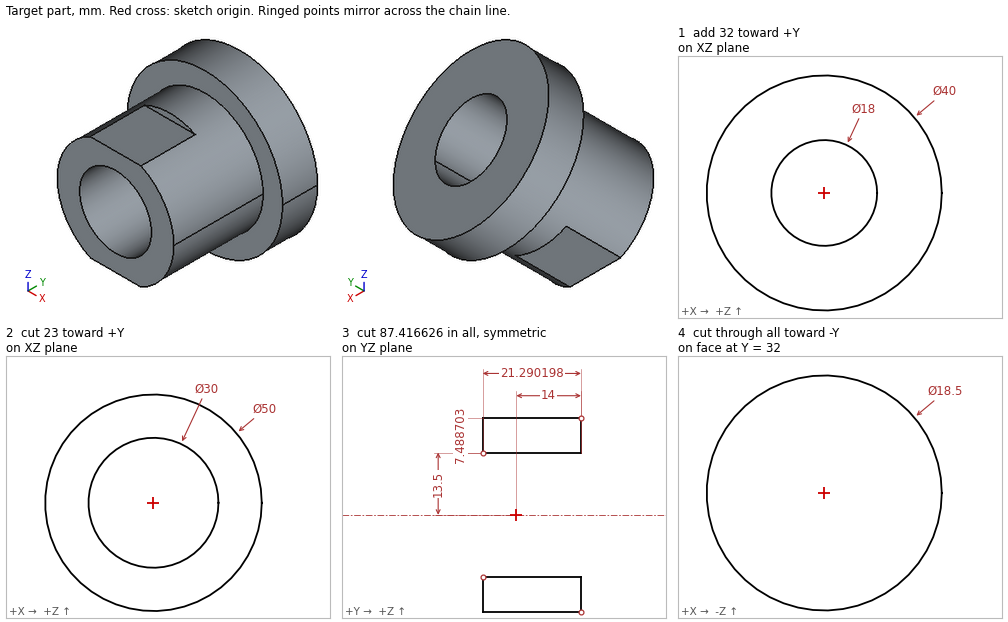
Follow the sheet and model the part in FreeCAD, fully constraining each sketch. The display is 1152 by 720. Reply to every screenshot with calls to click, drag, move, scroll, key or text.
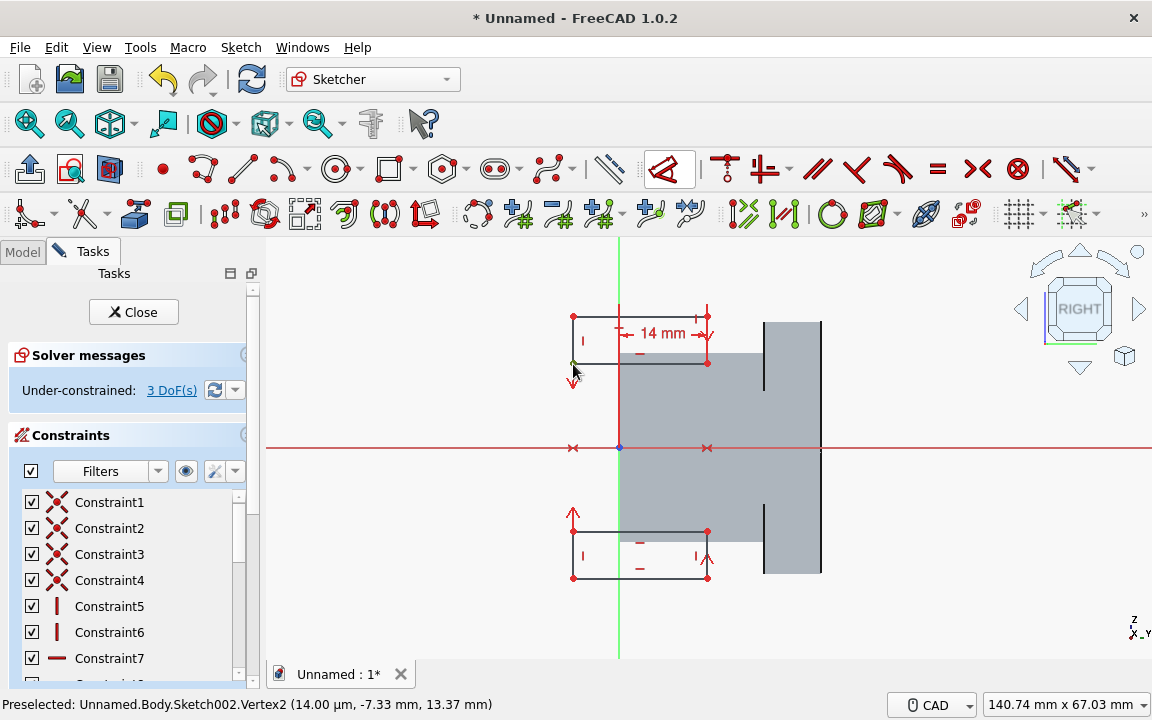
key(i)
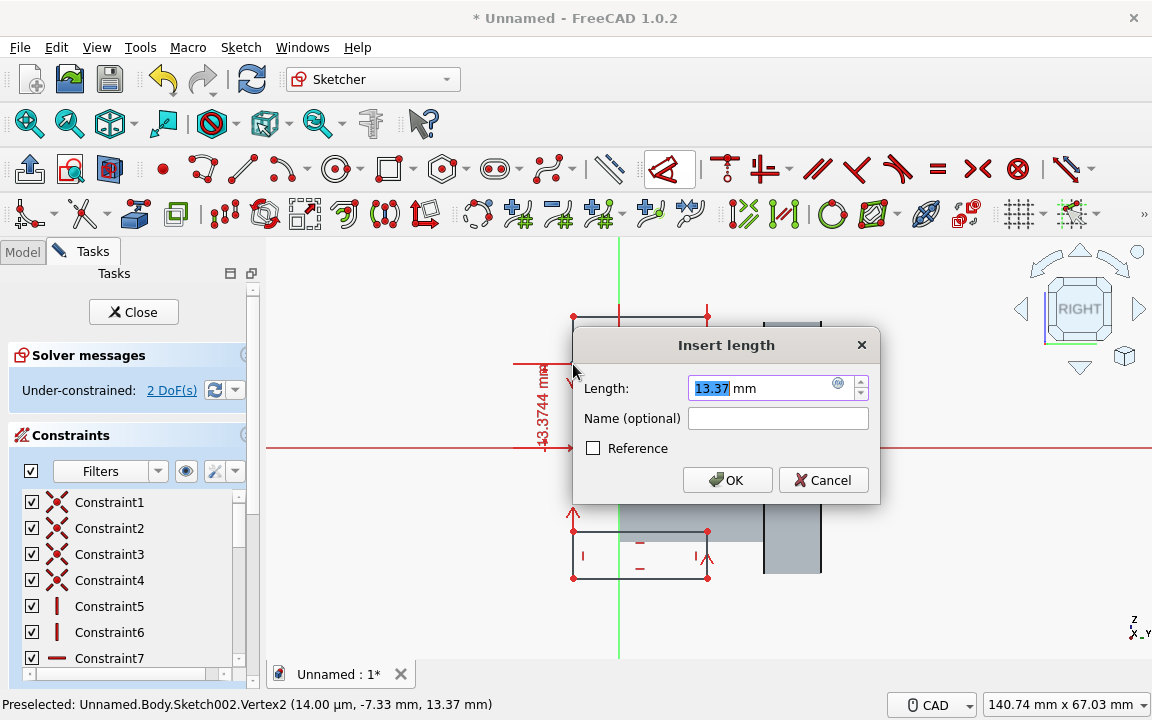
text(13.5)
key(Return)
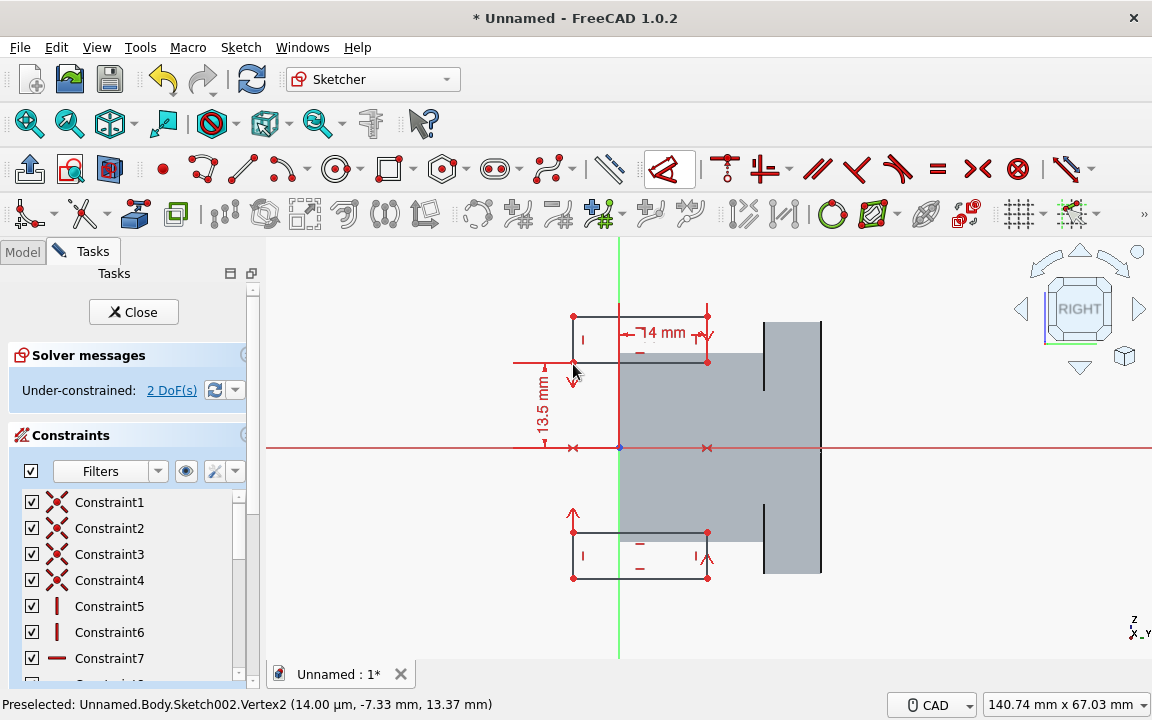
click(573, 330)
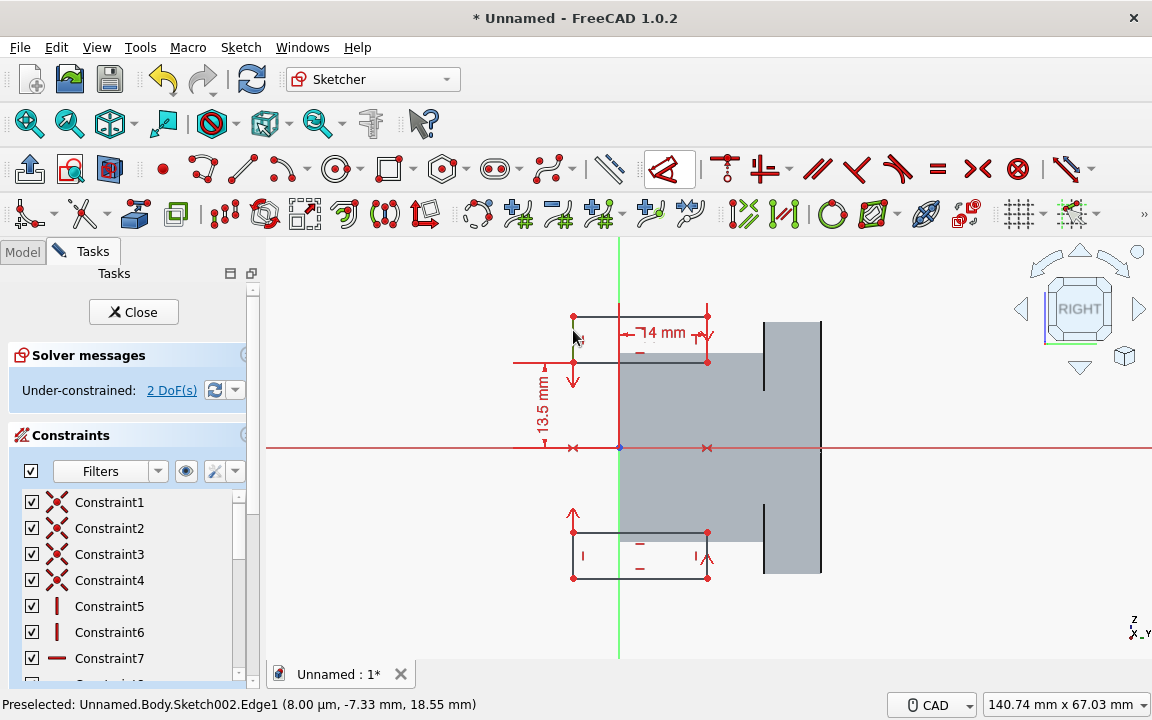
key(i)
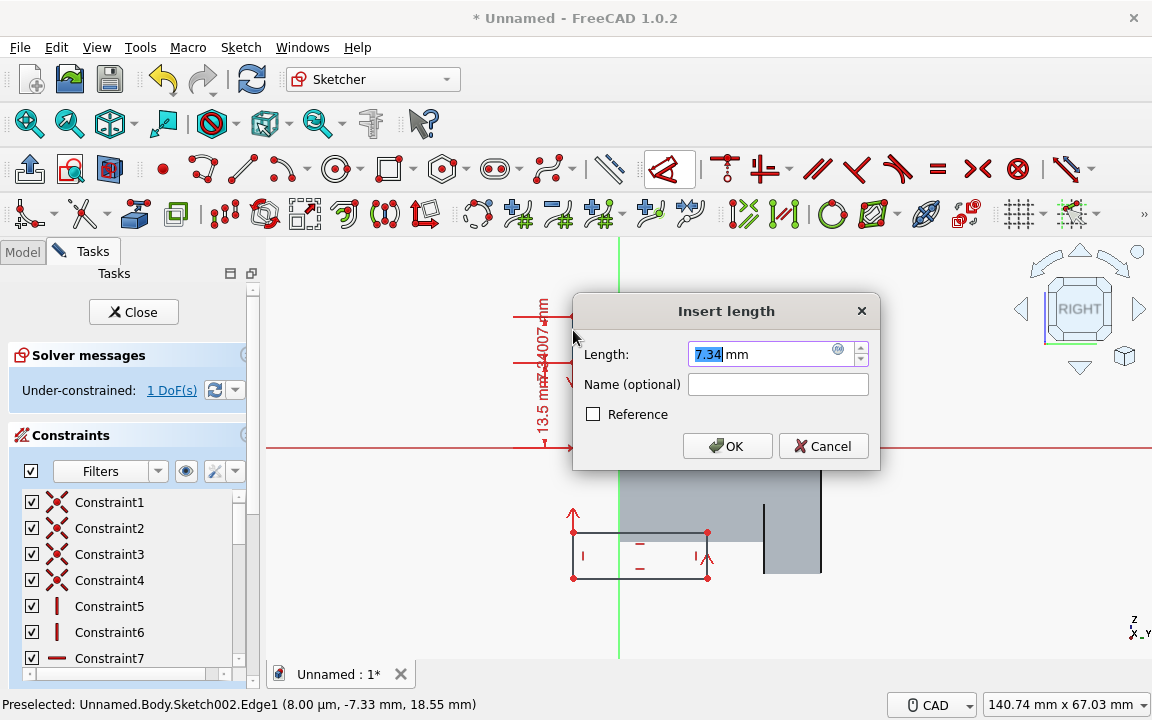
text(7.488703)
key(Return)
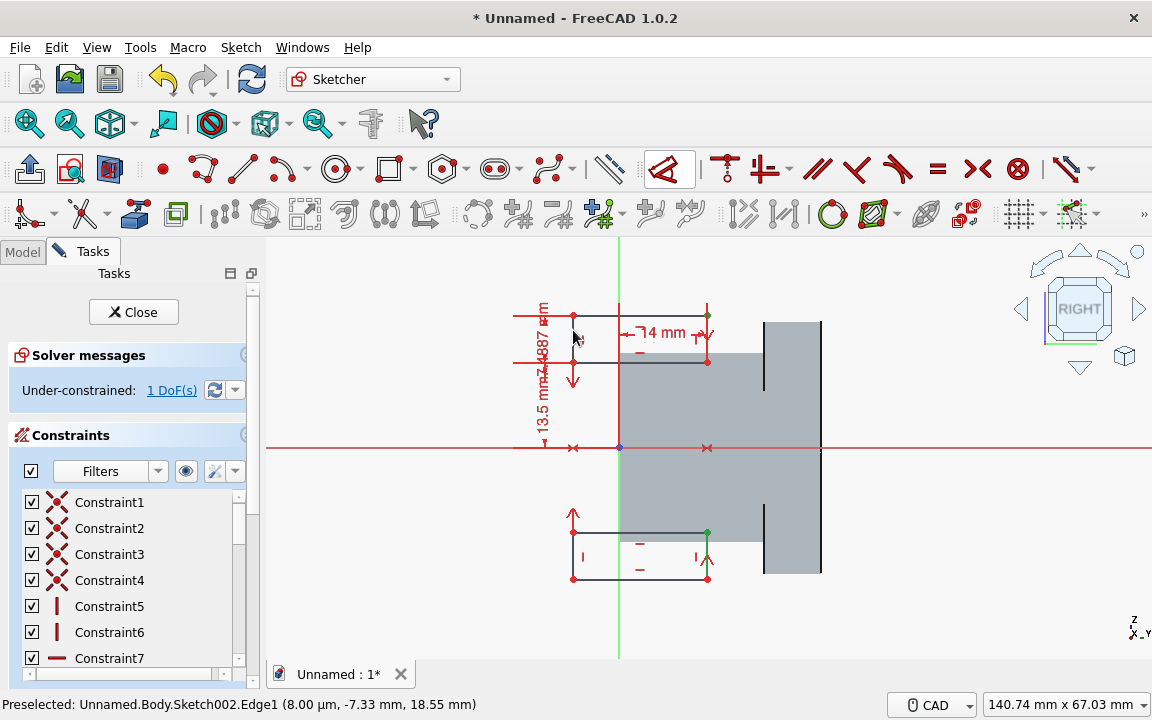
click(667, 363)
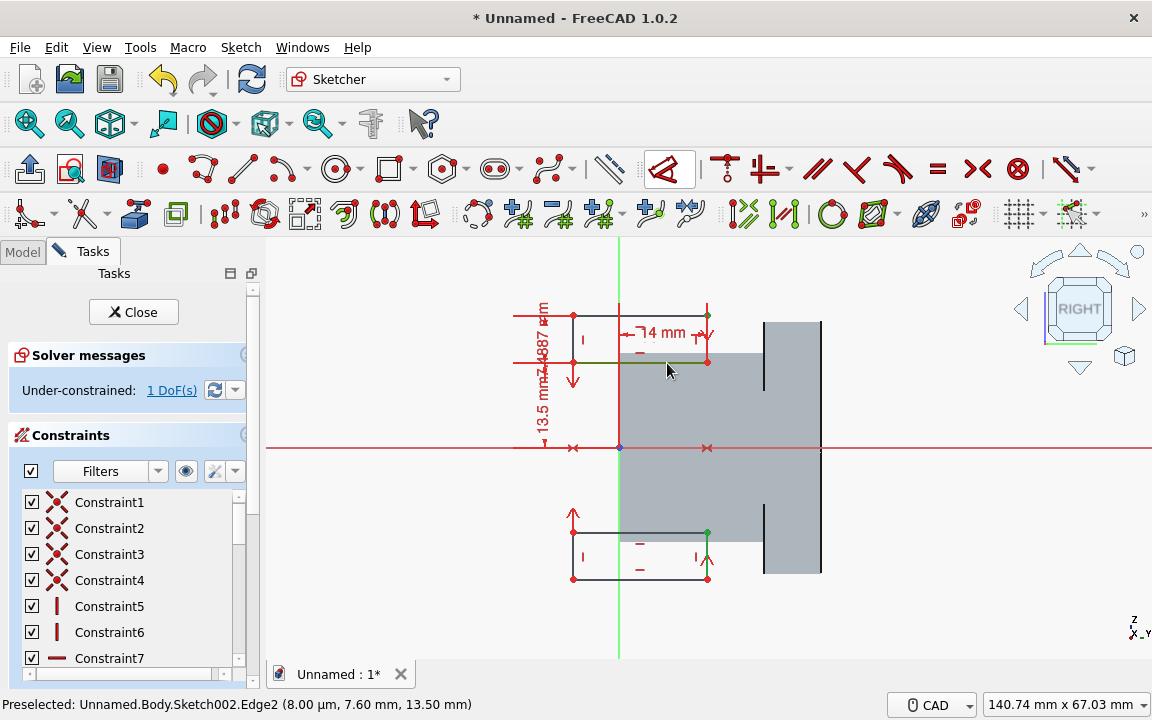
key(l)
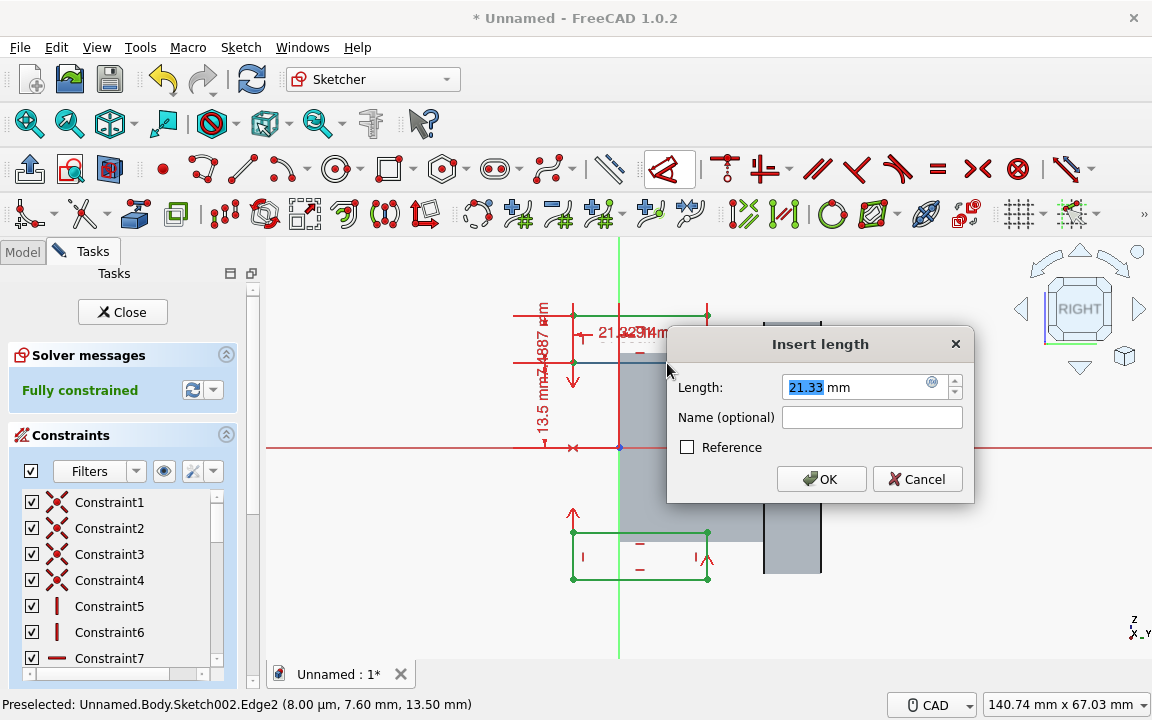
text(21.290198)
key(Return)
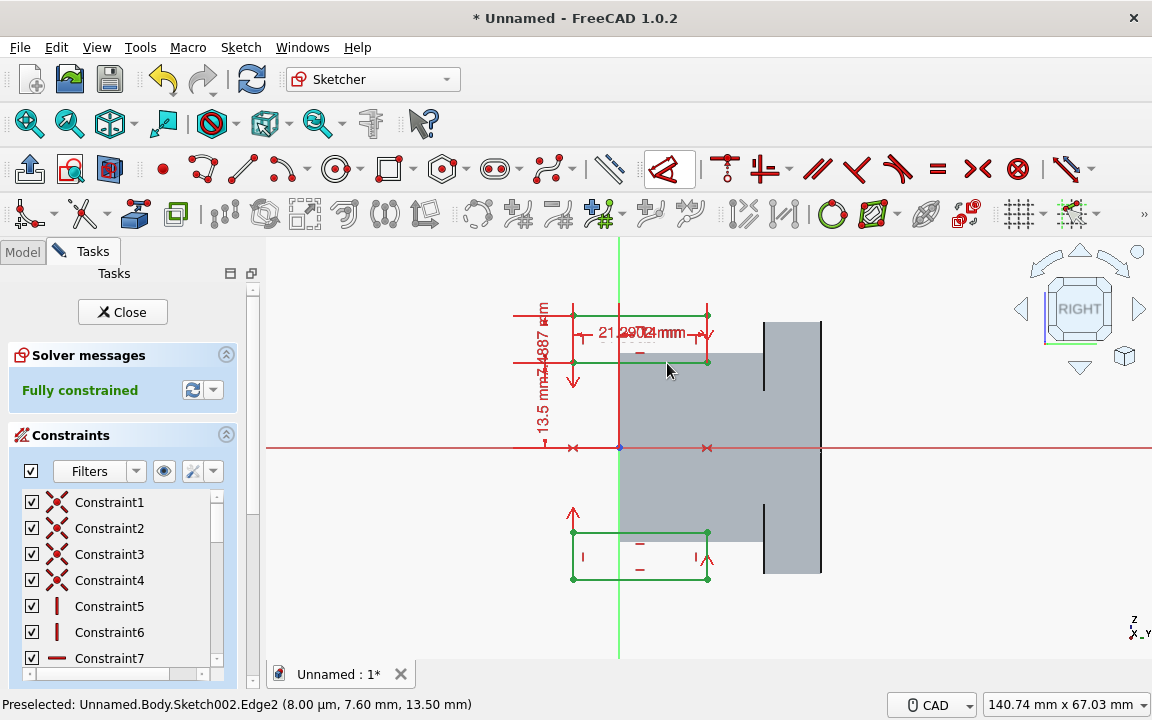
click(123, 312)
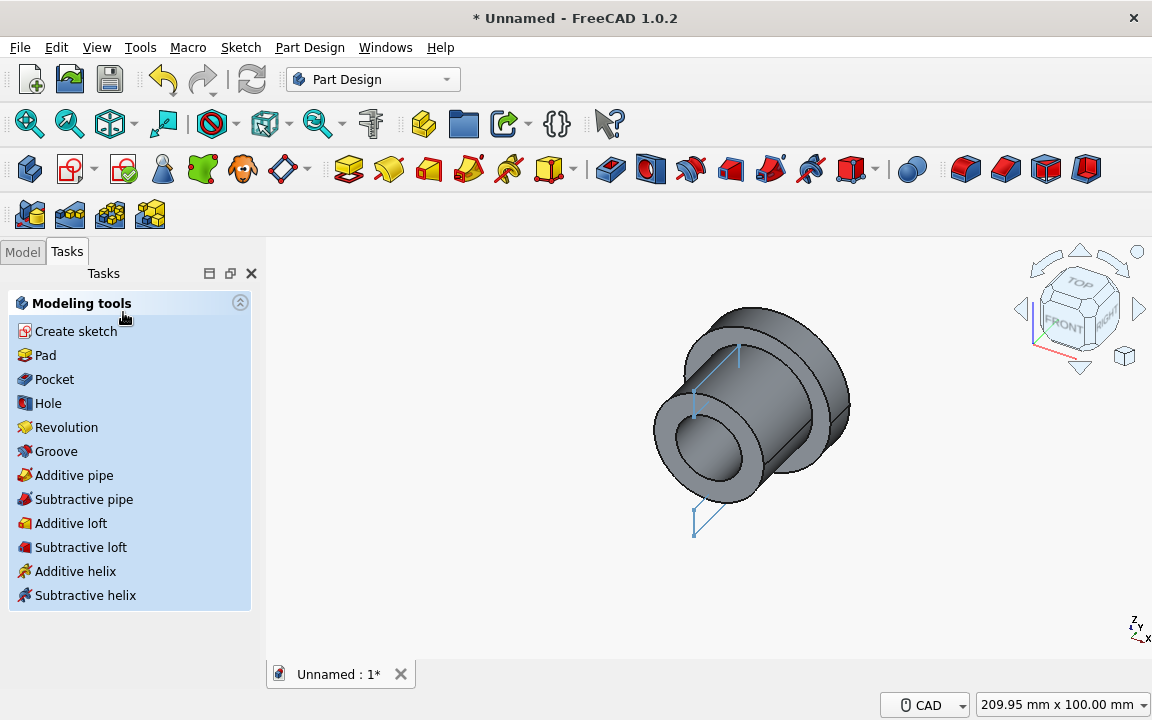
click(612, 170)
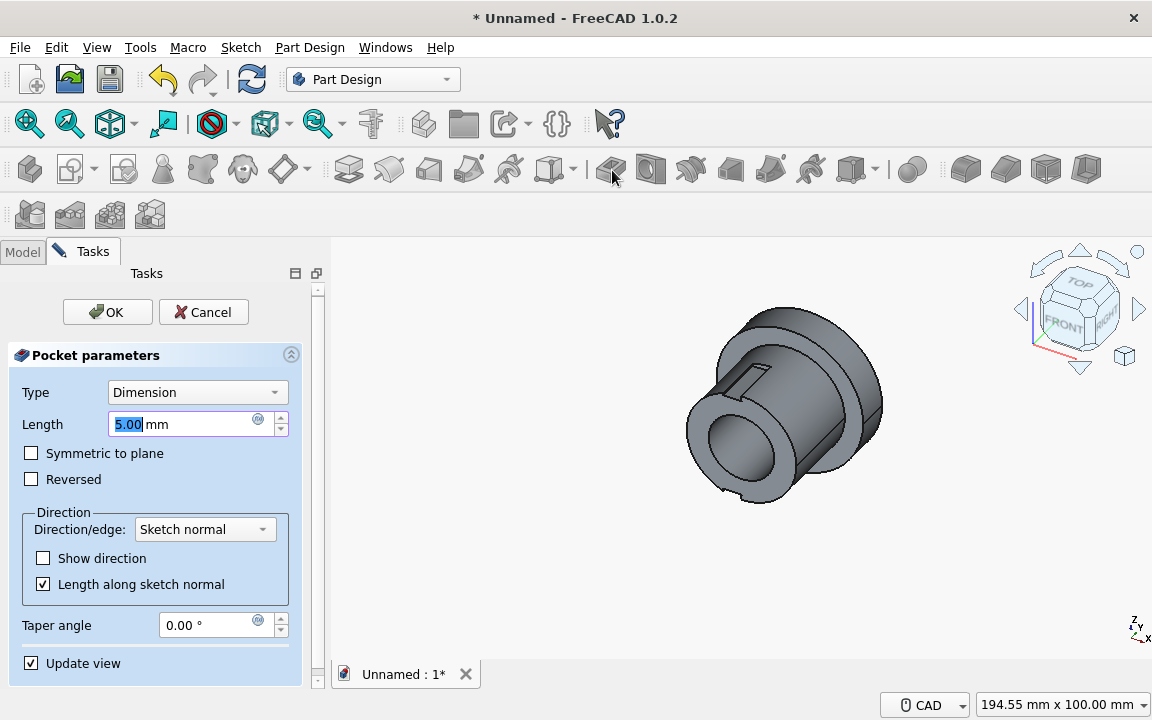
text(87.416626)
key(Tab)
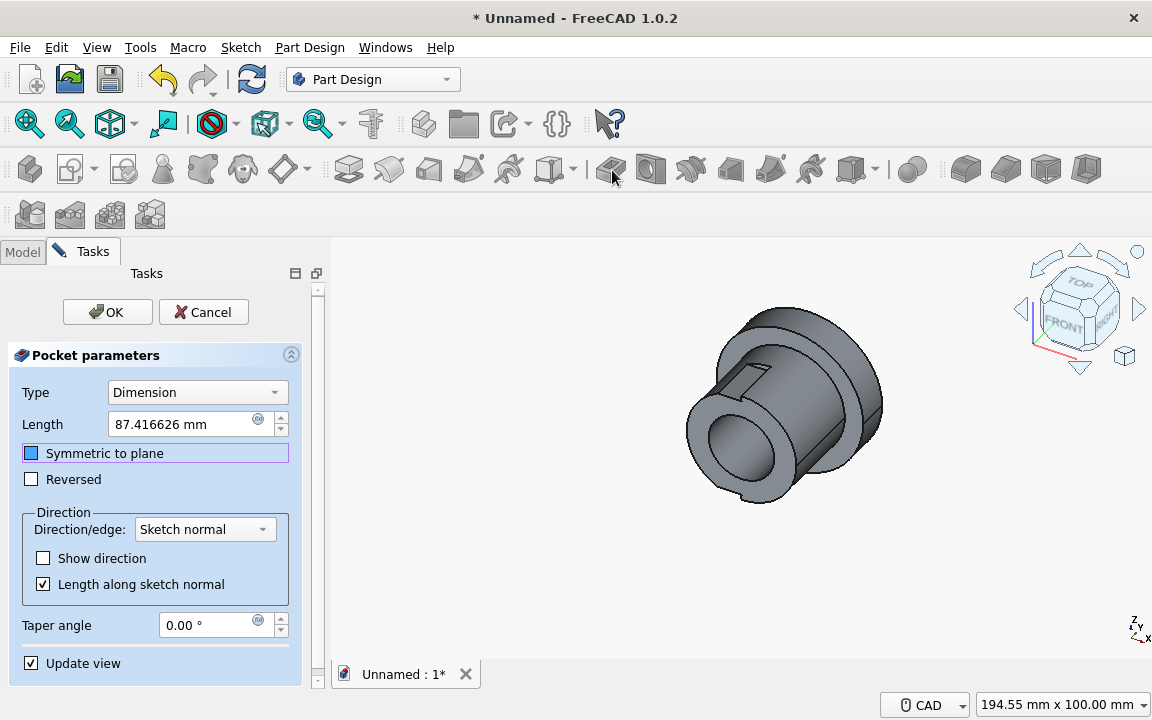
click(30, 453)